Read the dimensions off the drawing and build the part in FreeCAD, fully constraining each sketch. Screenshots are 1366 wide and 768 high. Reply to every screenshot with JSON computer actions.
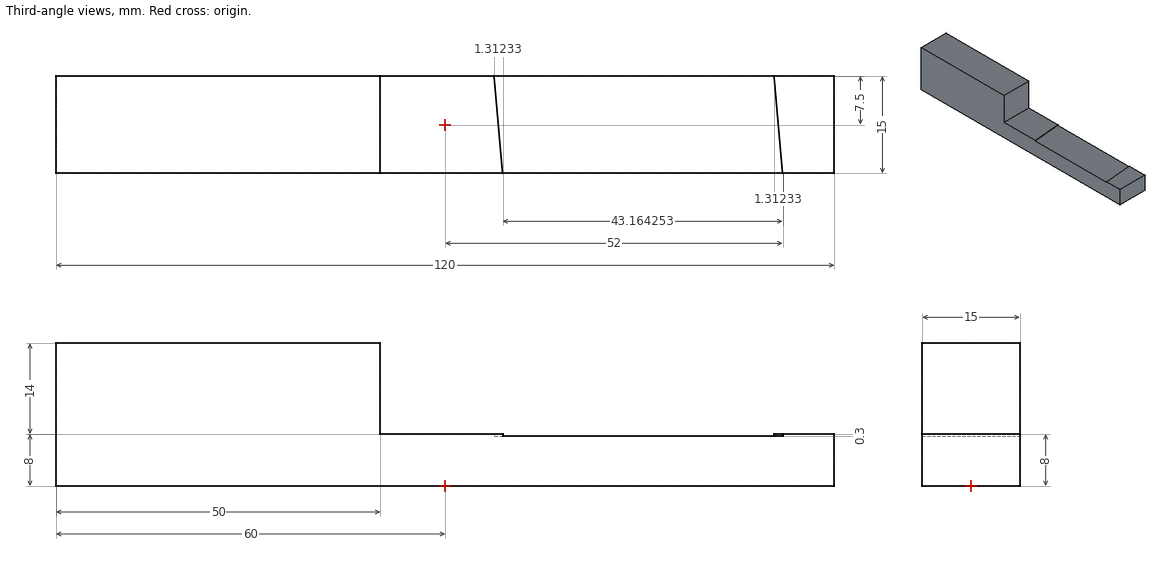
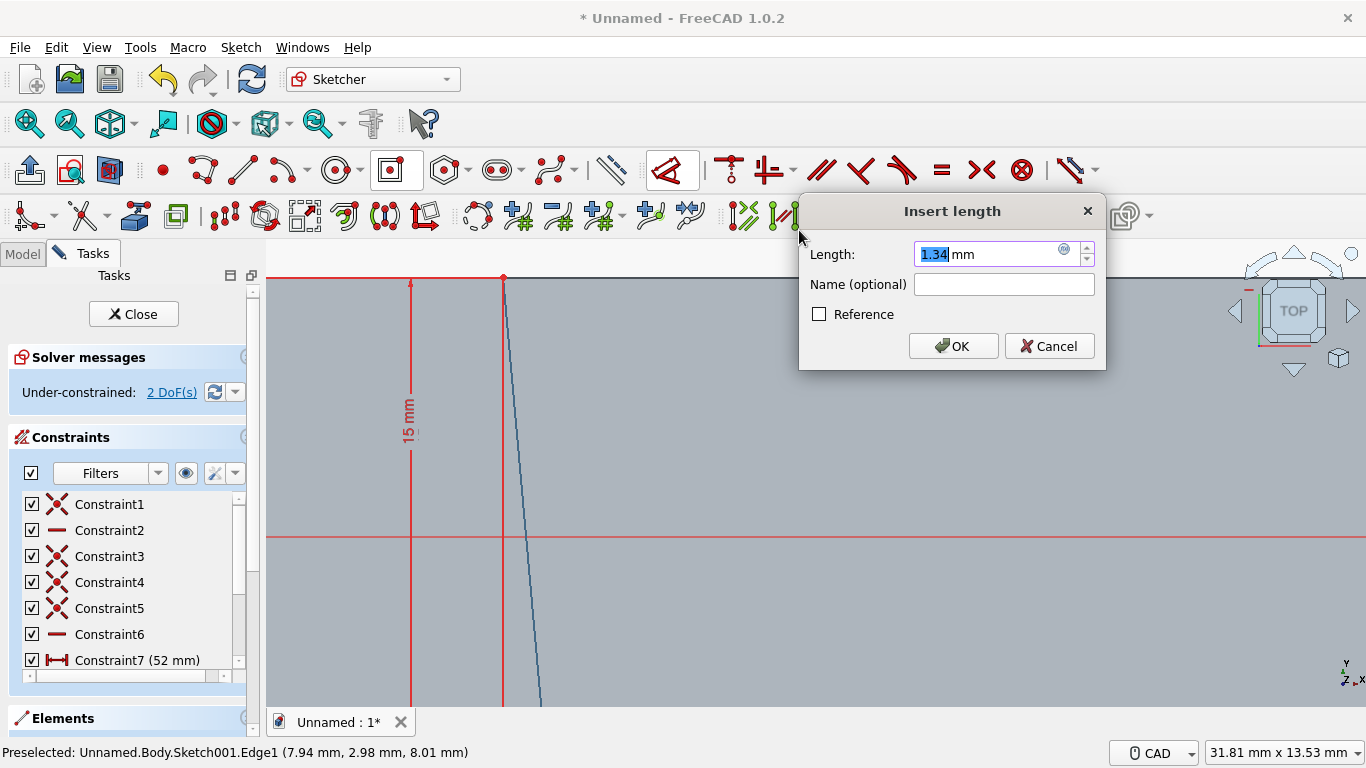
{"action": "type", "text": "1.31233"}
{"action": "key", "text": "Return"}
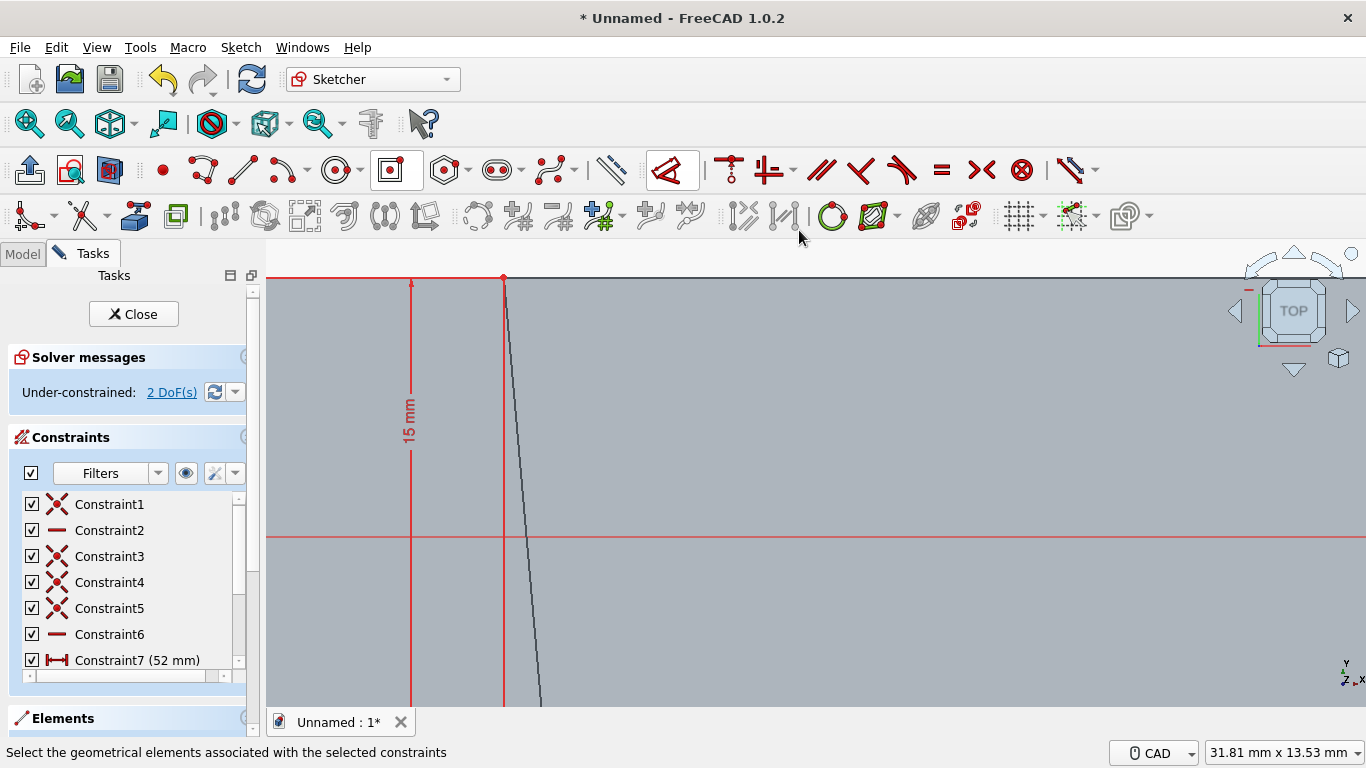
{"action": "scroll", "coordinate": [518, 436], "scroll_direction": "down", "scroll_amount": 5}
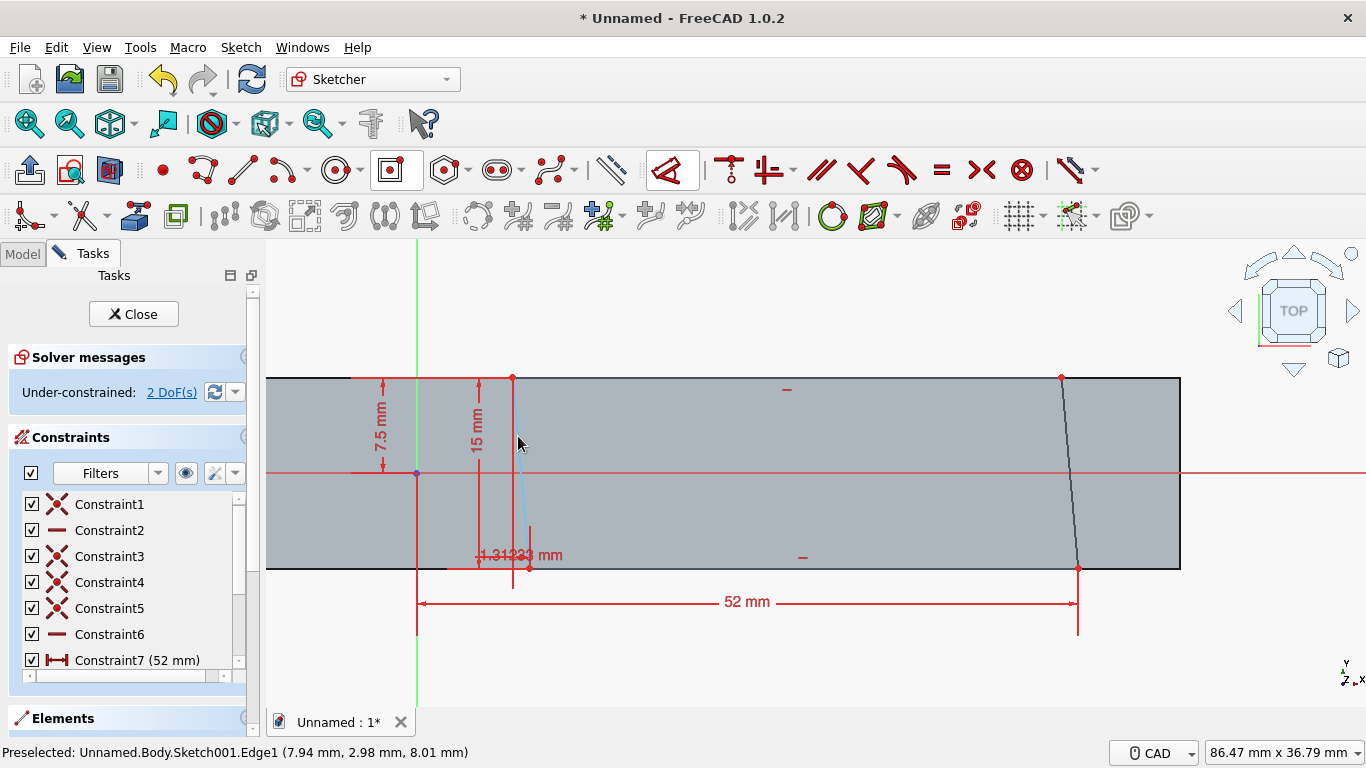
{"action": "scroll", "coordinate": [1073, 512], "scroll_direction": "up", "scroll_amount": 5}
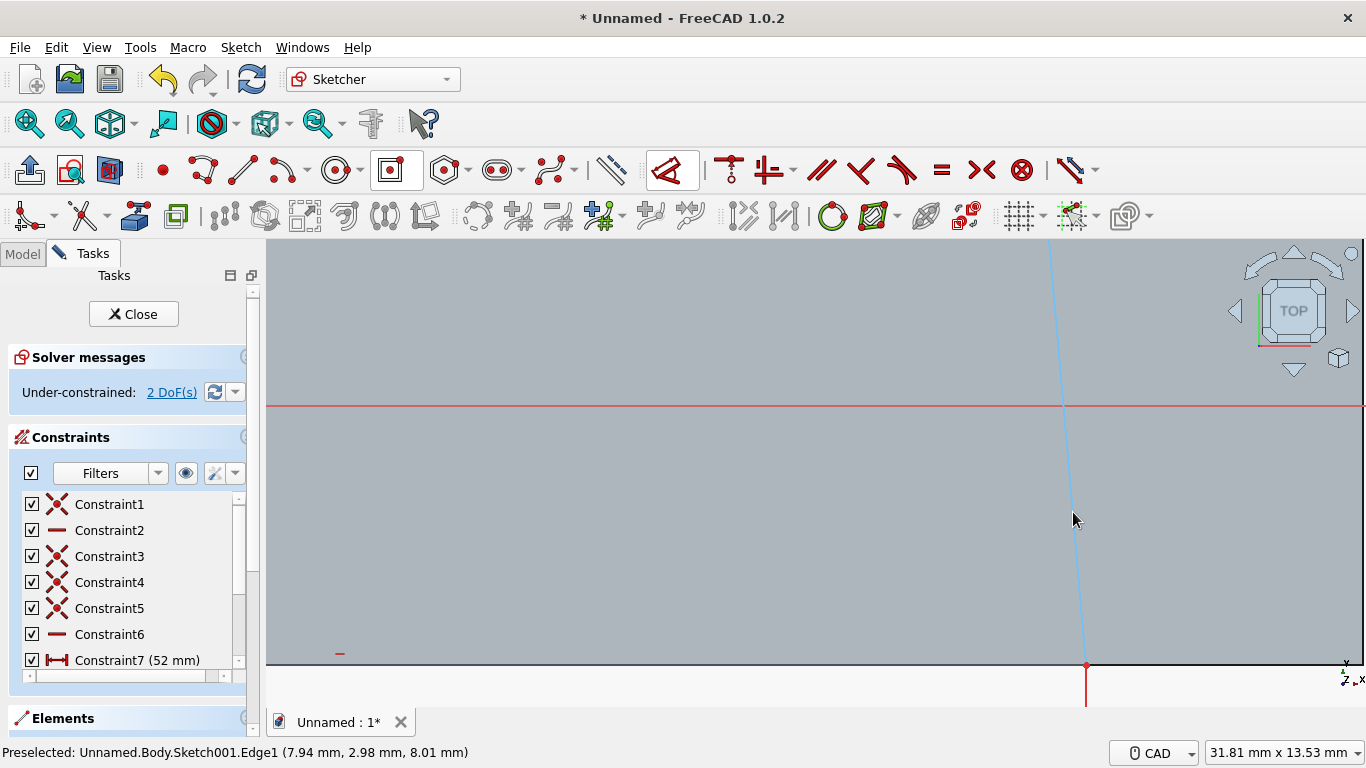
{"action": "left_click", "coordinate": [1073, 510]}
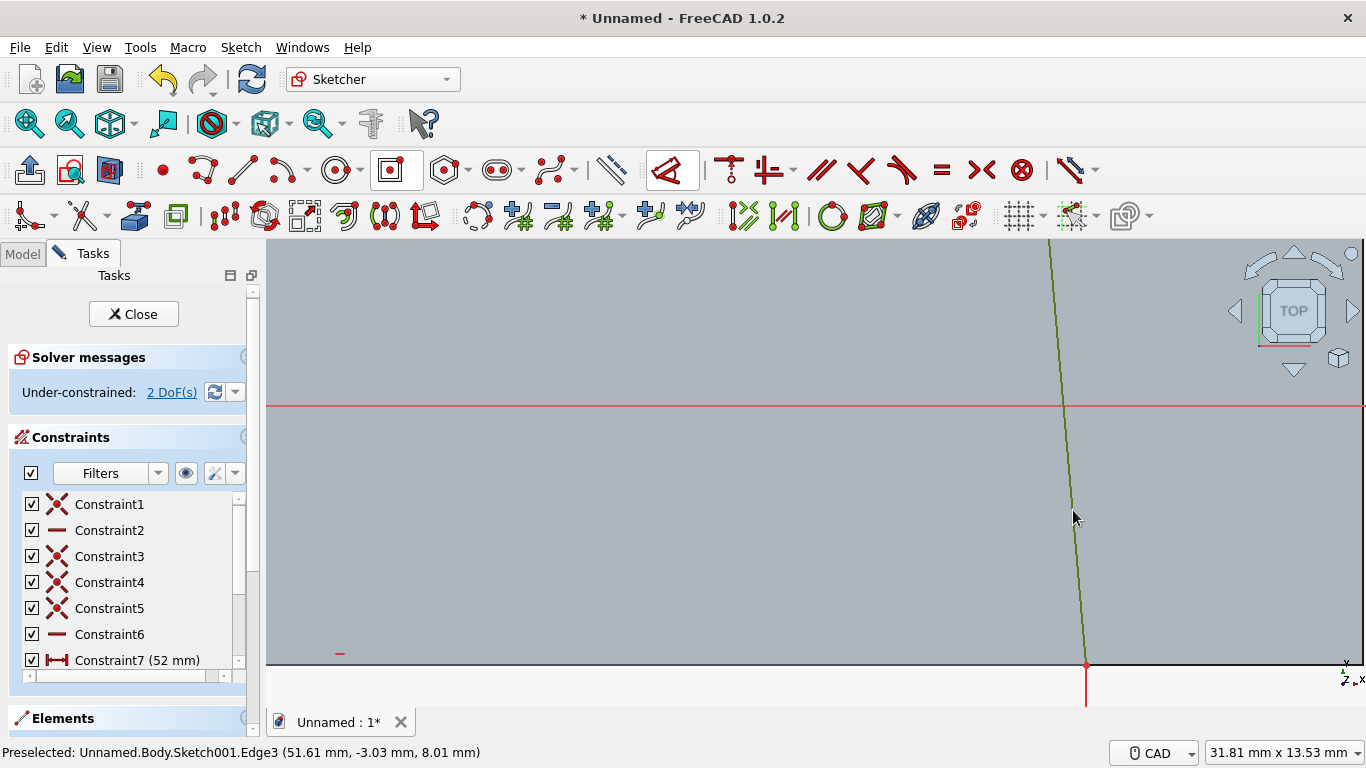
{"action": "left_click", "coordinate": [694, 170]}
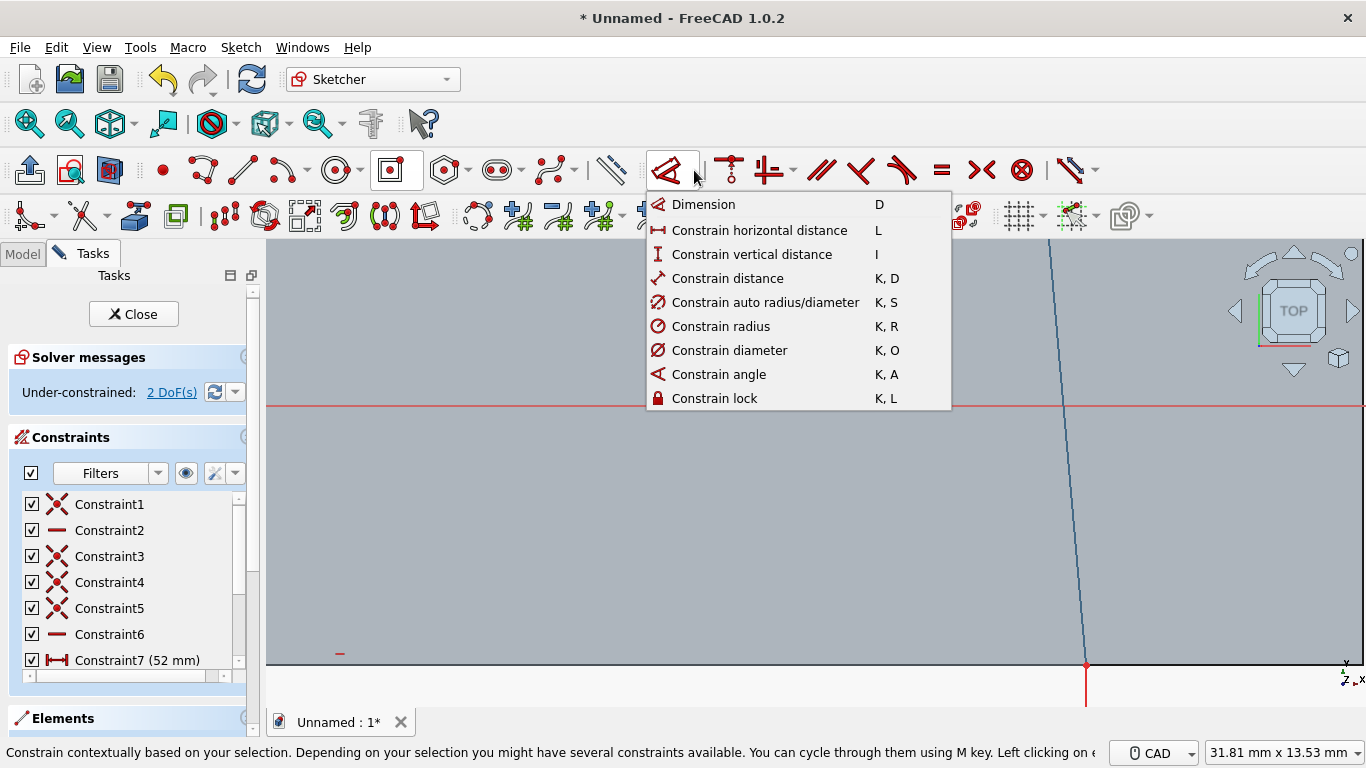
{"action": "left_click", "coordinate": [799, 230]}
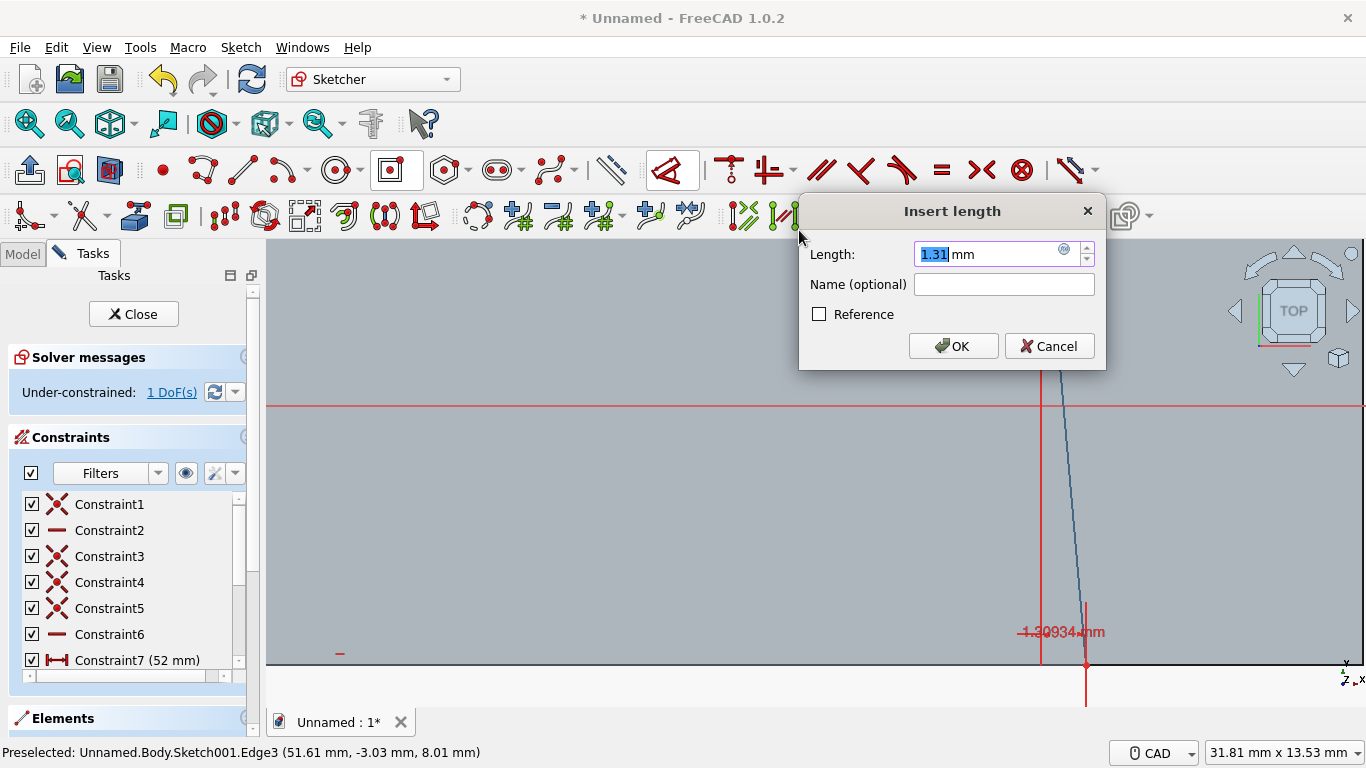
{"action": "type", "text": "1.31233"}
{"action": "key", "text": "Return"}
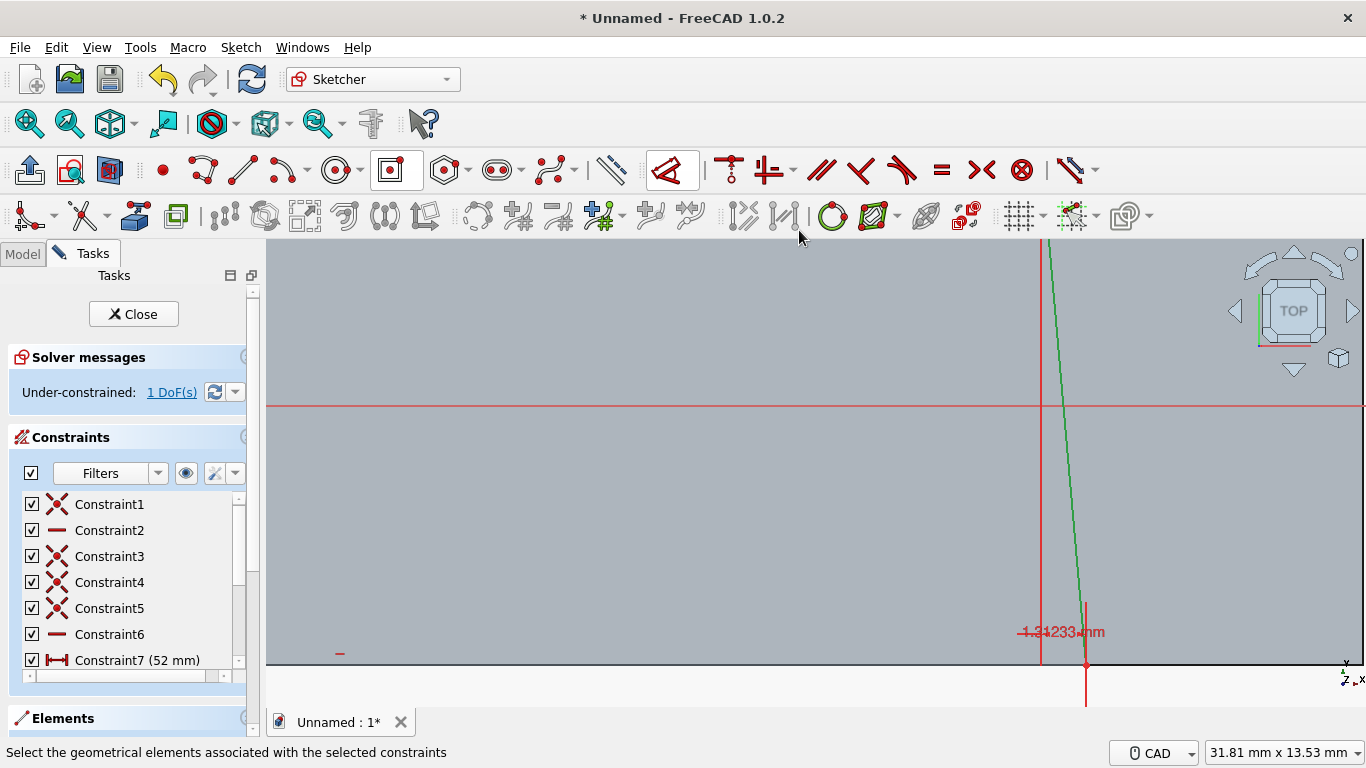
{"action": "left_click", "coordinate": [639, 665]}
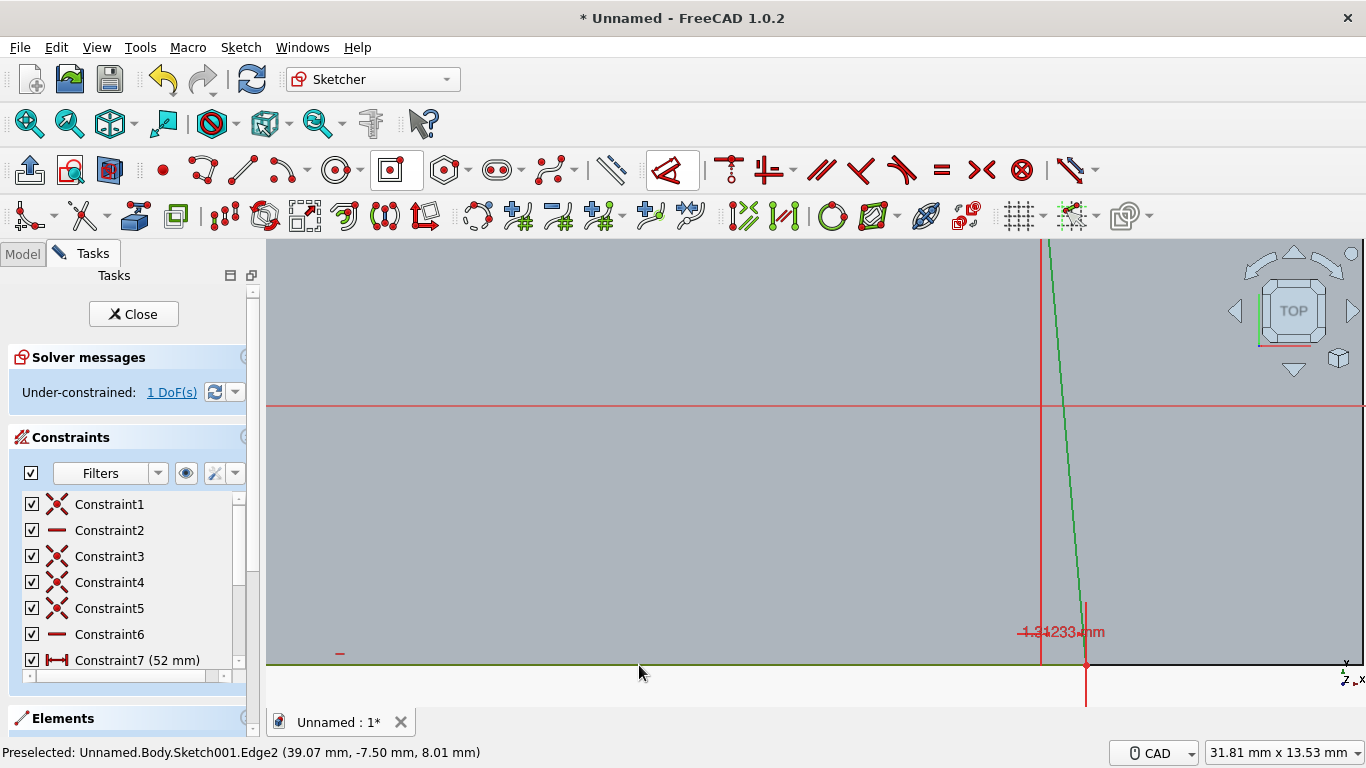
{"action": "key", "text": "l"}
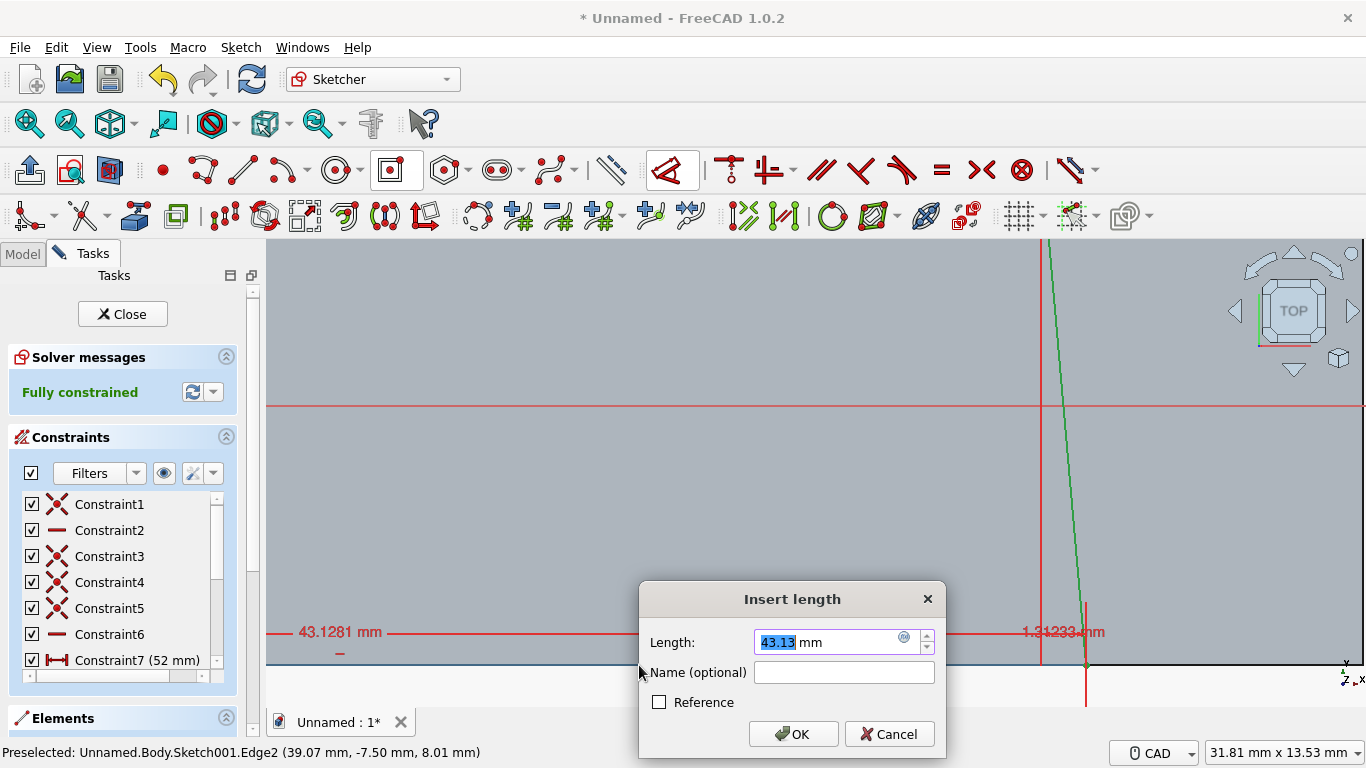
{"action": "type", "text": "43.164253"}
{"action": "key", "text": "Return"}